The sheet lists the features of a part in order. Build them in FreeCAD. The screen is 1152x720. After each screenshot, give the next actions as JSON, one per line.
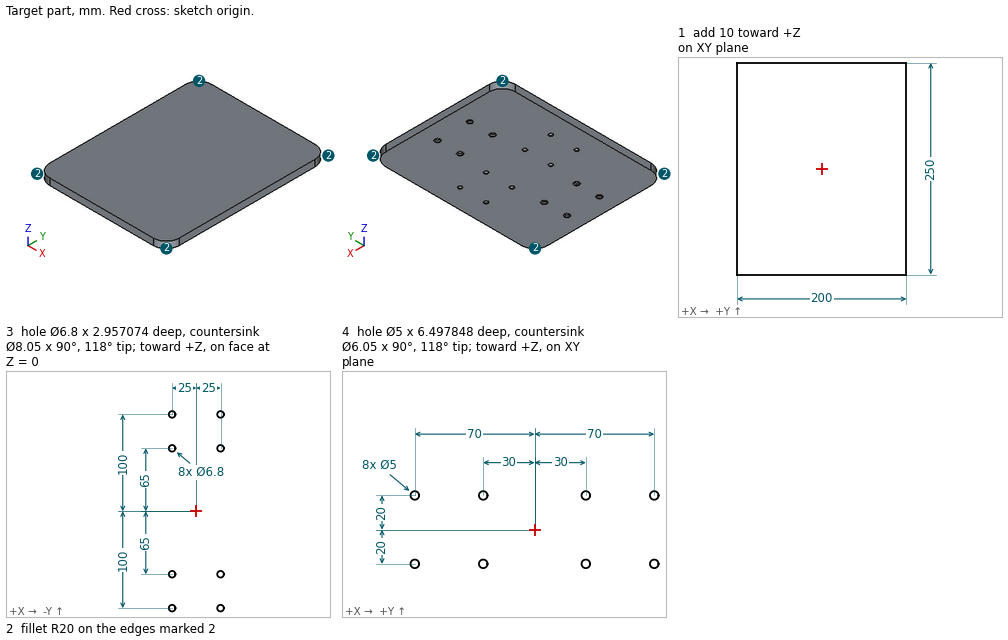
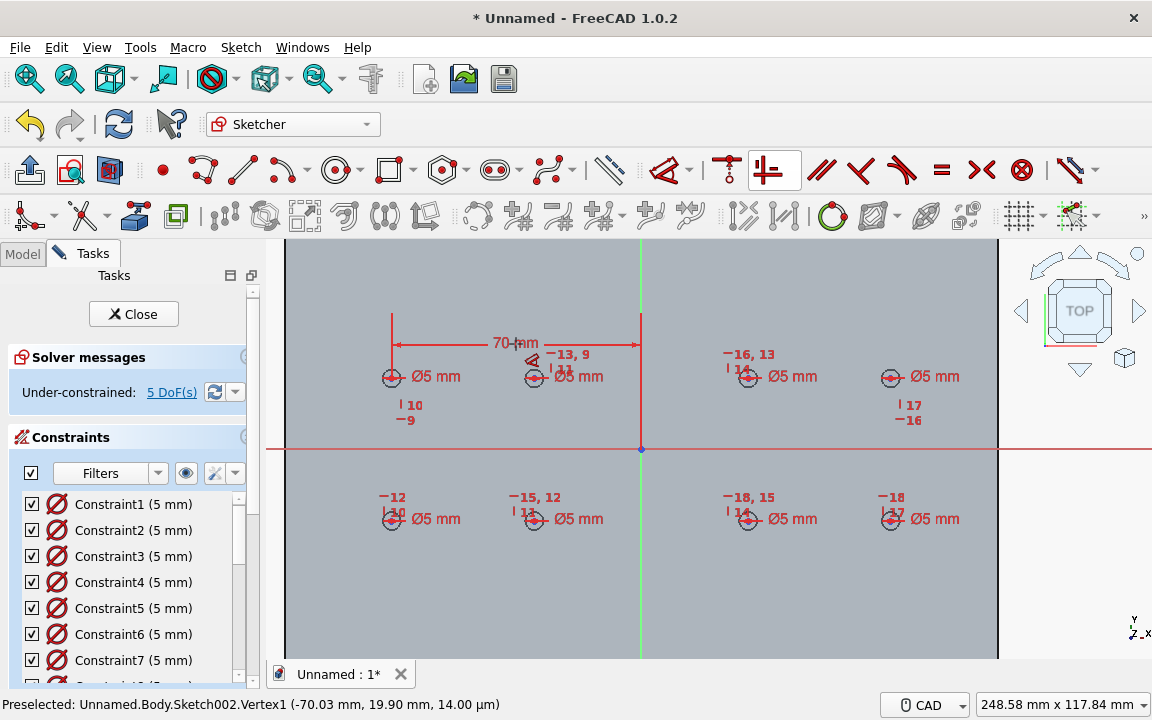
{"action": "left_click", "coordinate": [392, 378]}
{"action": "left_click", "coordinate": [358, 414]}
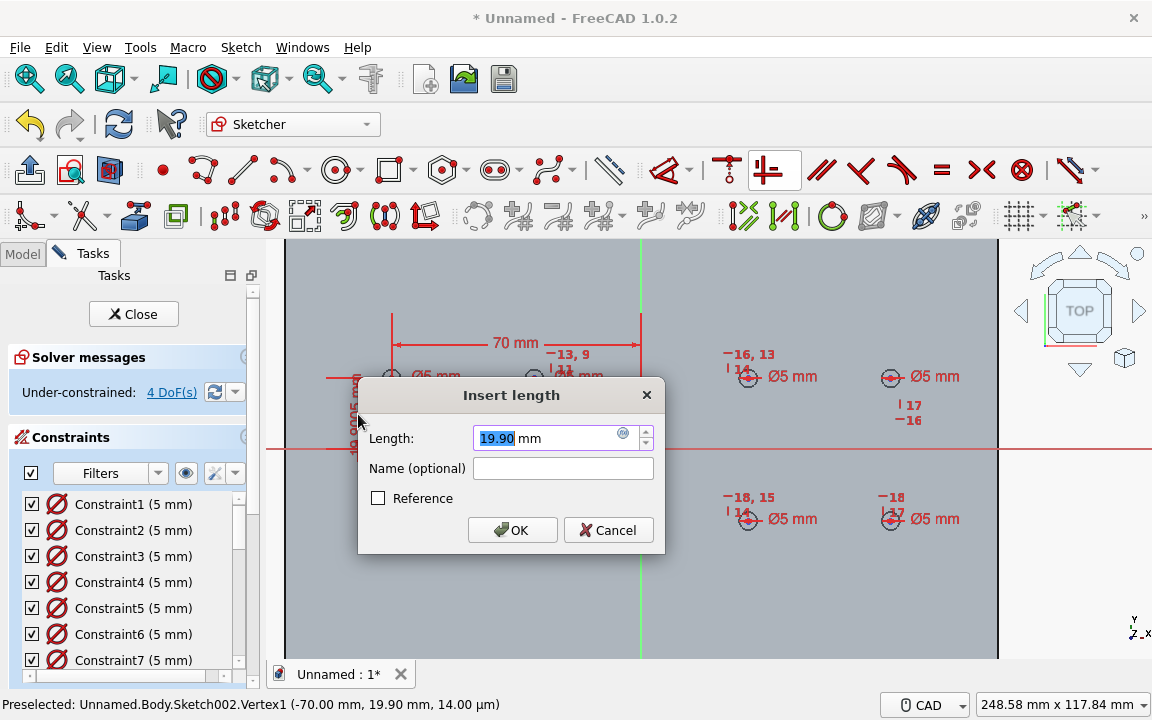
{"action": "type", "text": "20"}
{"action": "key", "text": "Return"}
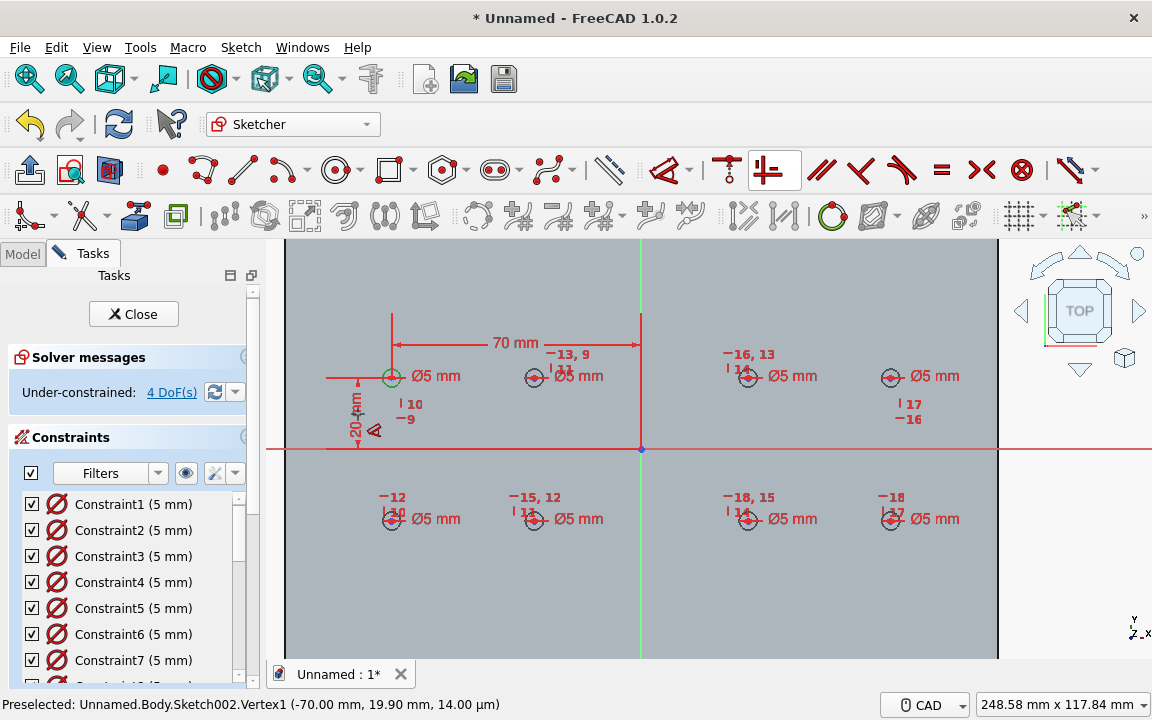
{"action": "left_click", "coordinate": [534, 378]}
{"action": "left_click", "coordinate": [588, 344]}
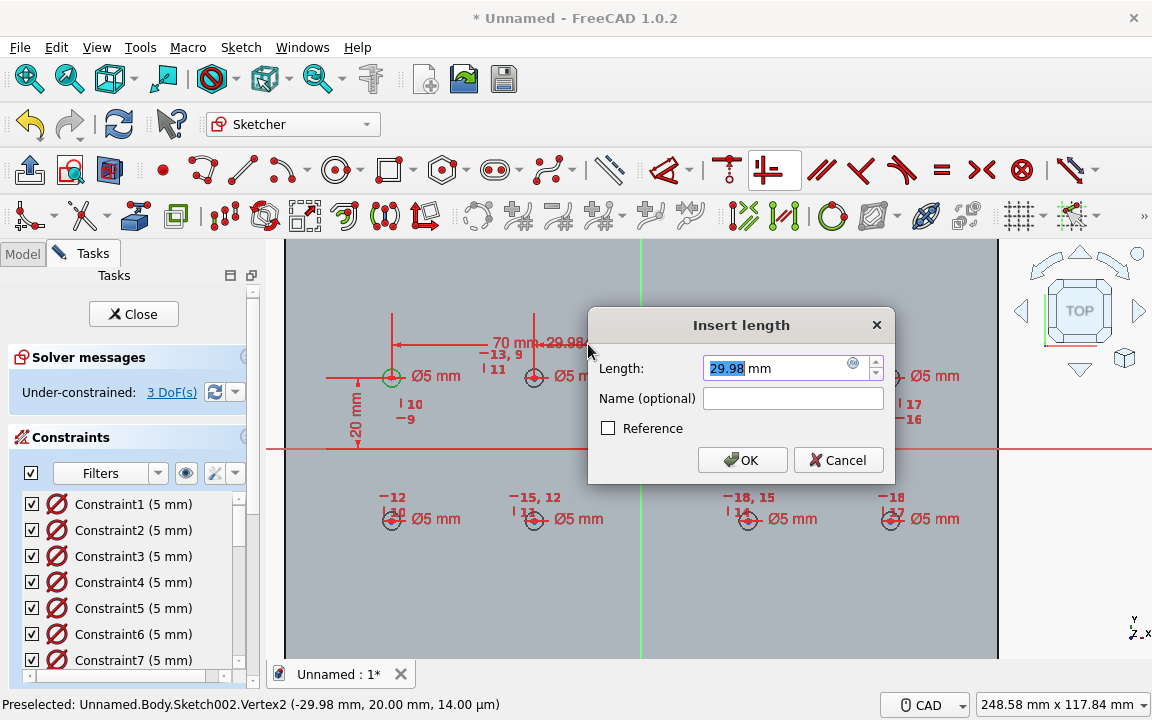
{"action": "type", "text": "30"}
{"action": "key", "text": "Return"}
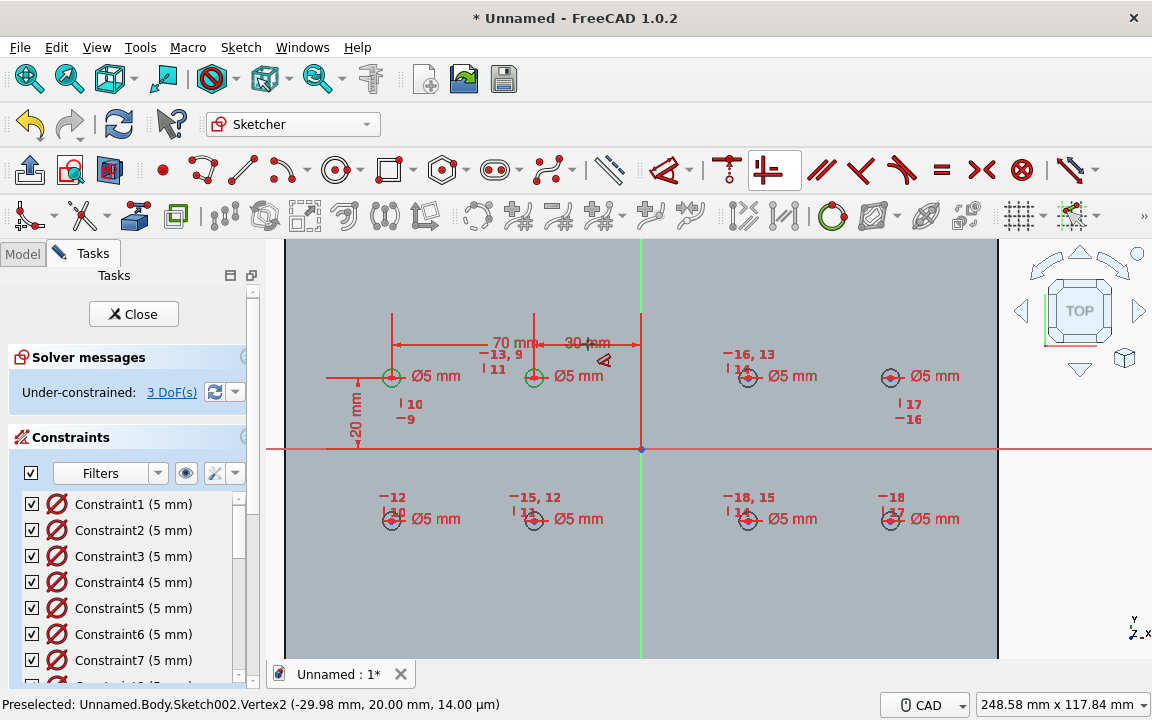
{"action": "left_click", "coordinate": [392, 521]}
{"action": "left_click", "coordinate": [358, 485]}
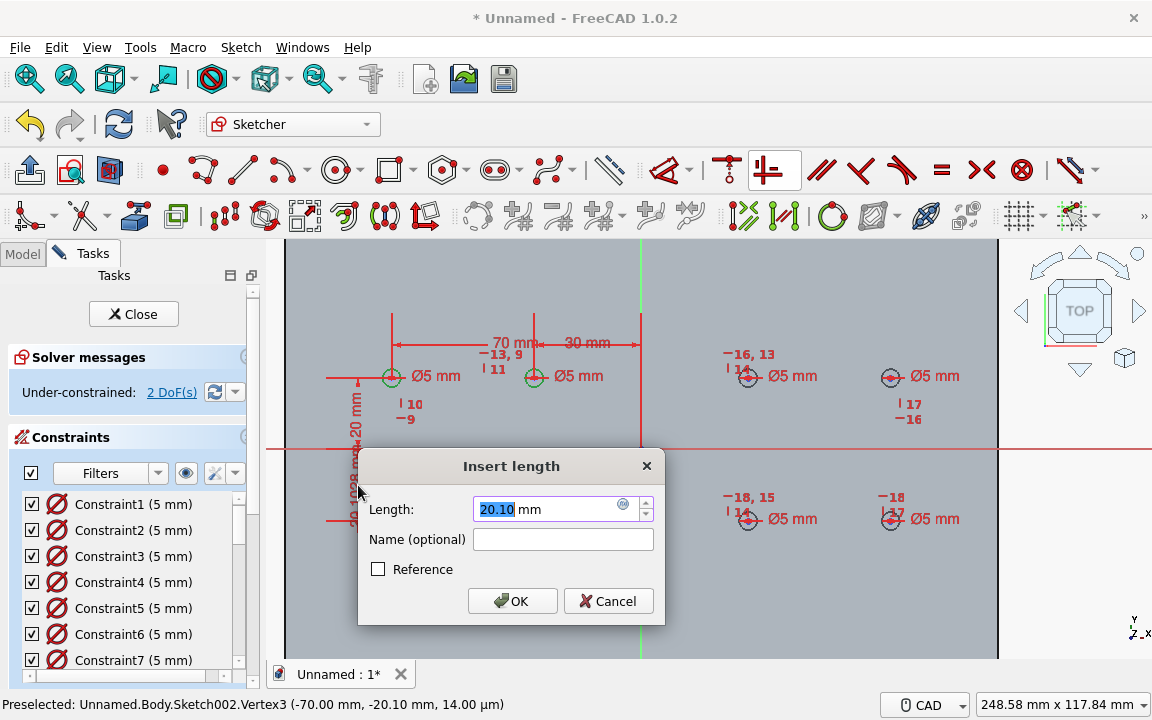
{"action": "type", "text": "20"}
{"action": "key", "text": "Return"}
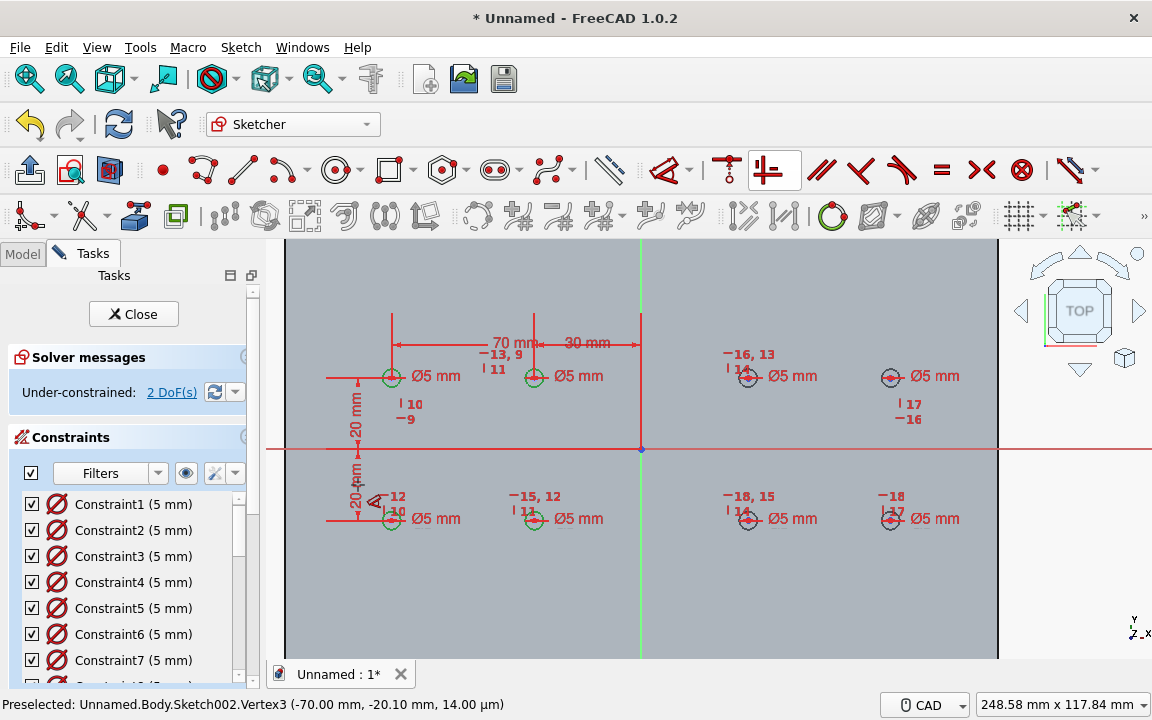
{"action": "left_click", "coordinate": [748, 378]}
{"action": "left_click", "coordinate": [695, 344]}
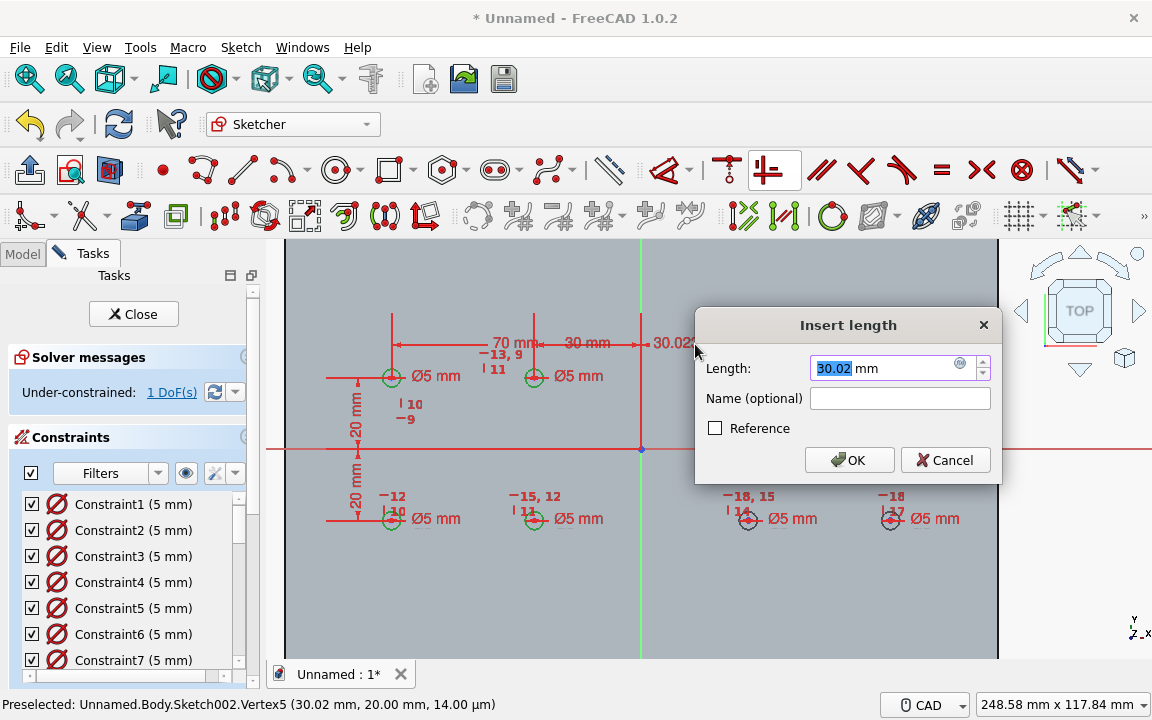
{"action": "type", "text": "30"}
{"action": "key", "text": "Return"}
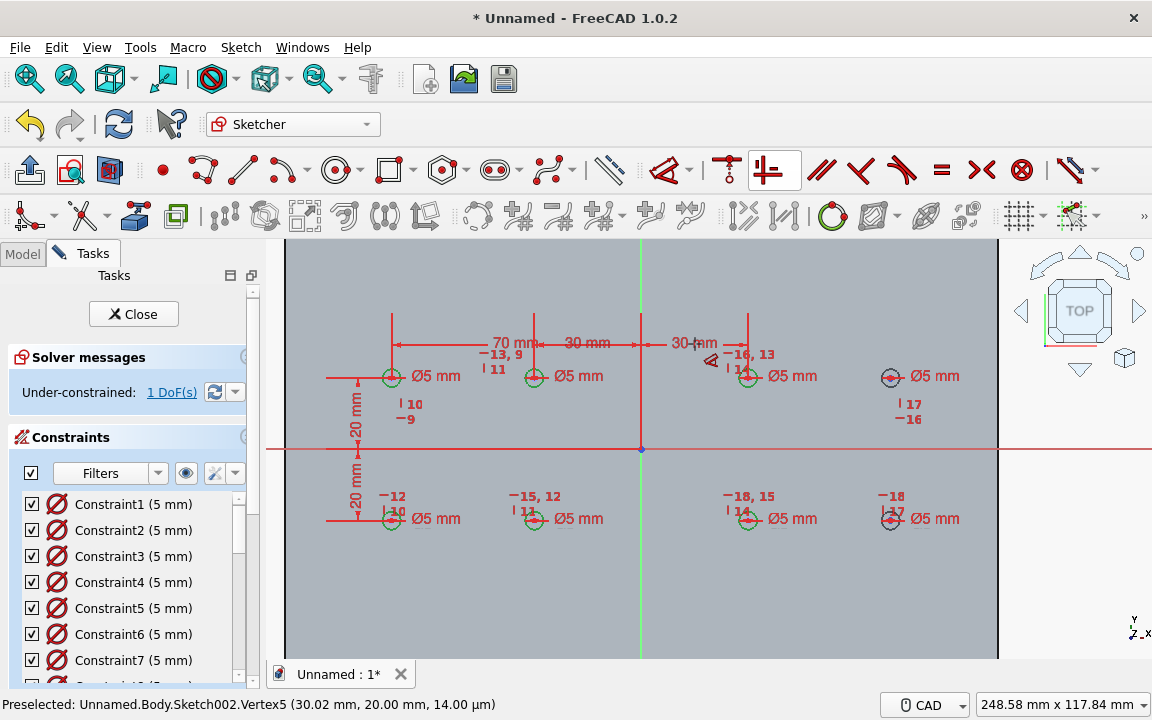
{"action": "left_click", "coordinate": [891, 378]}
{"action": "left_click", "coordinate": [766, 344]}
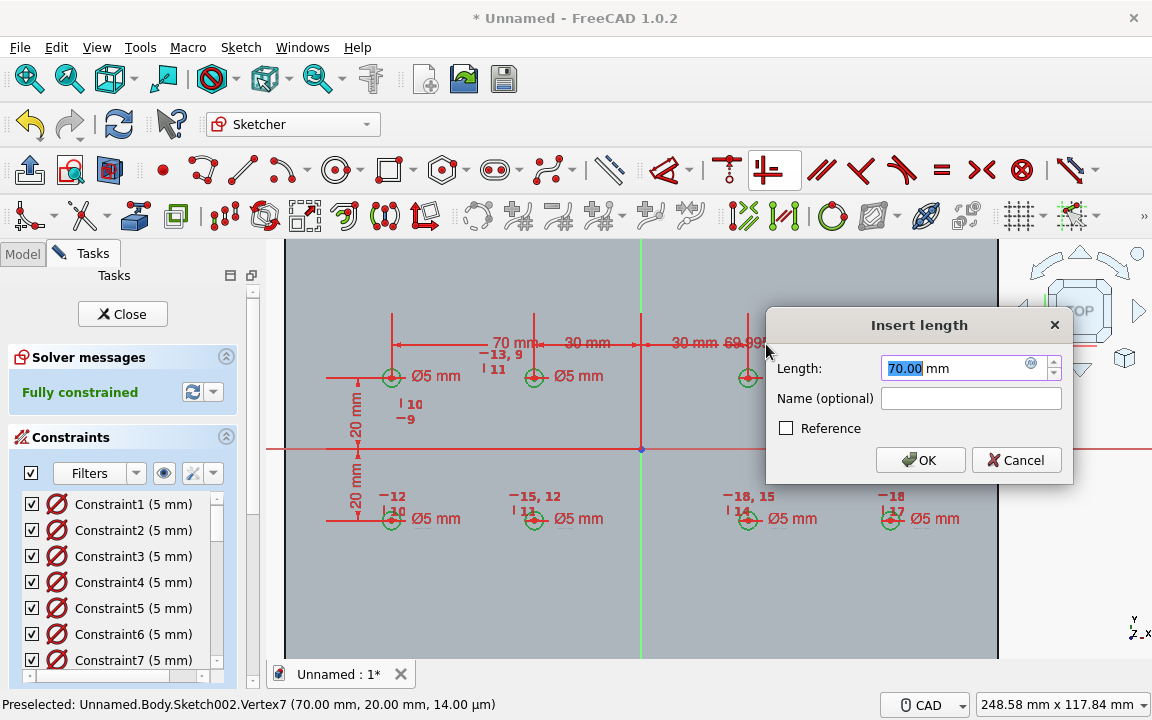
{"action": "type", "text": "70"}
{"action": "key", "text": "Return"}
{"action": "key", "text": "Escape"}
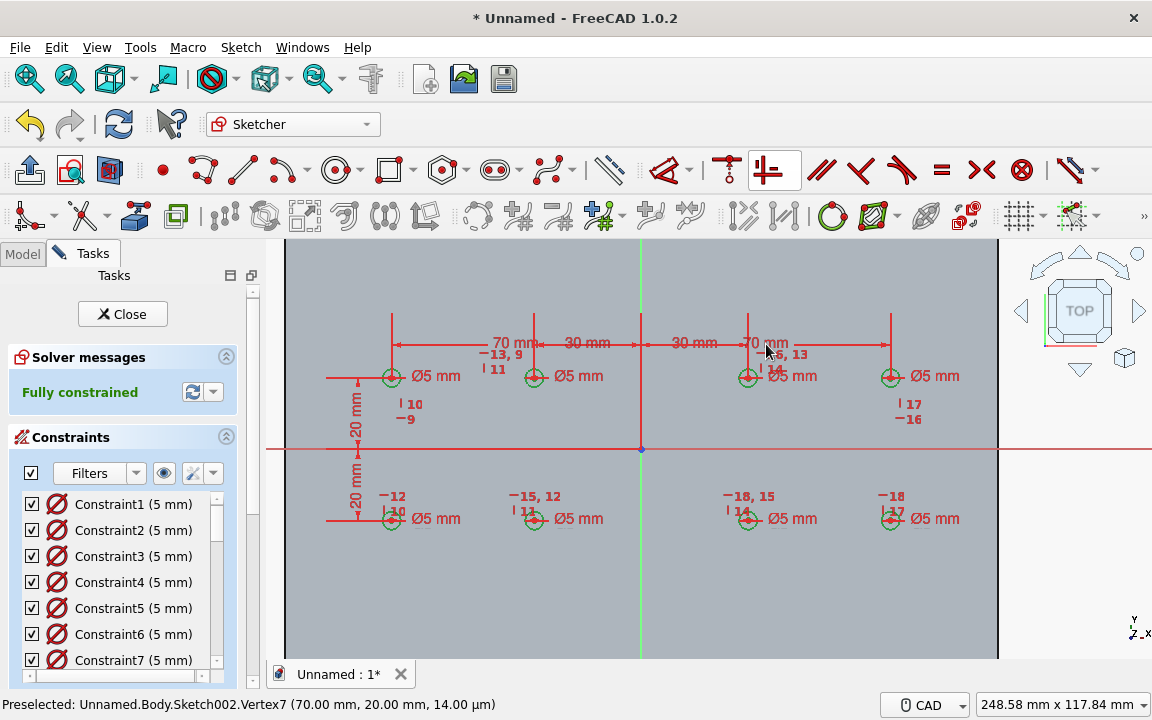
{"action": "left_click", "coordinate": [123, 314]}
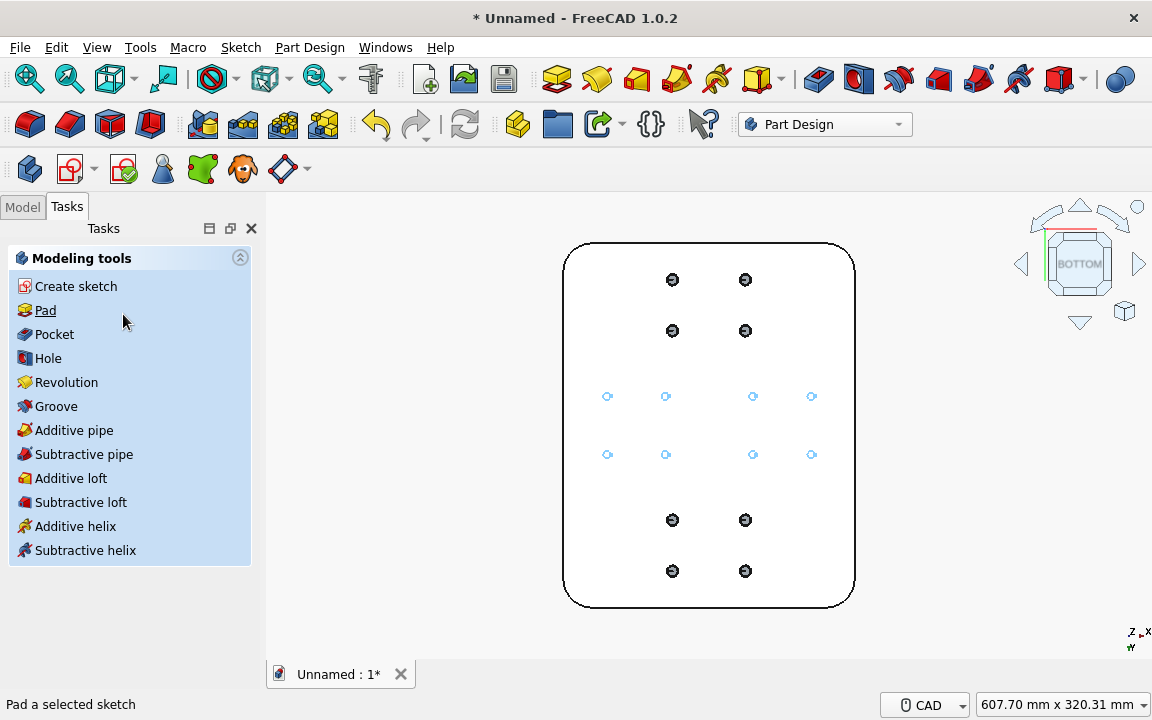
{"action": "left_click", "coordinate": [860, 80]}